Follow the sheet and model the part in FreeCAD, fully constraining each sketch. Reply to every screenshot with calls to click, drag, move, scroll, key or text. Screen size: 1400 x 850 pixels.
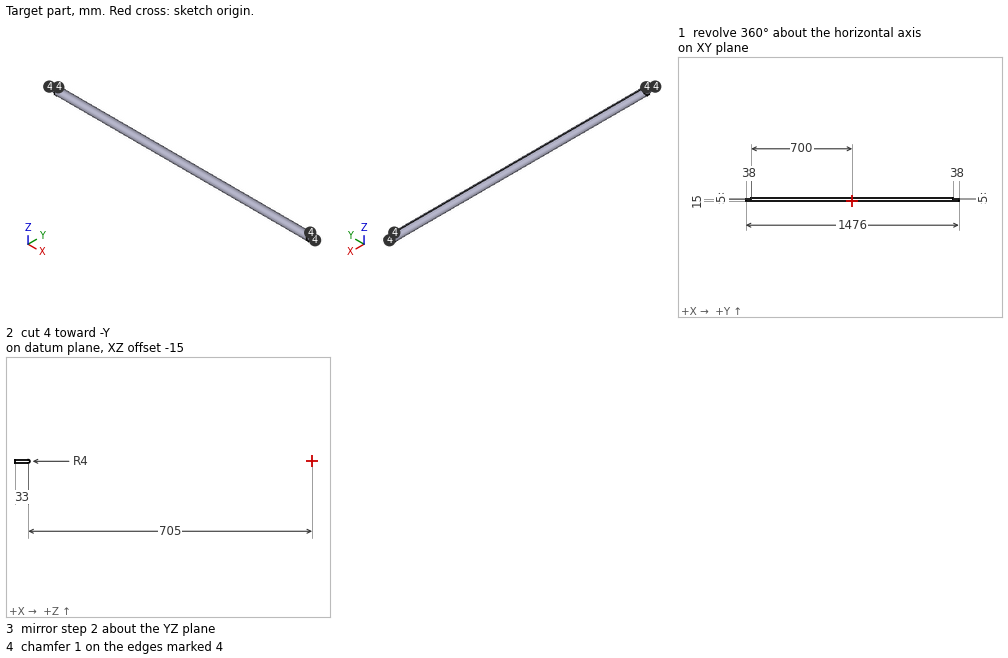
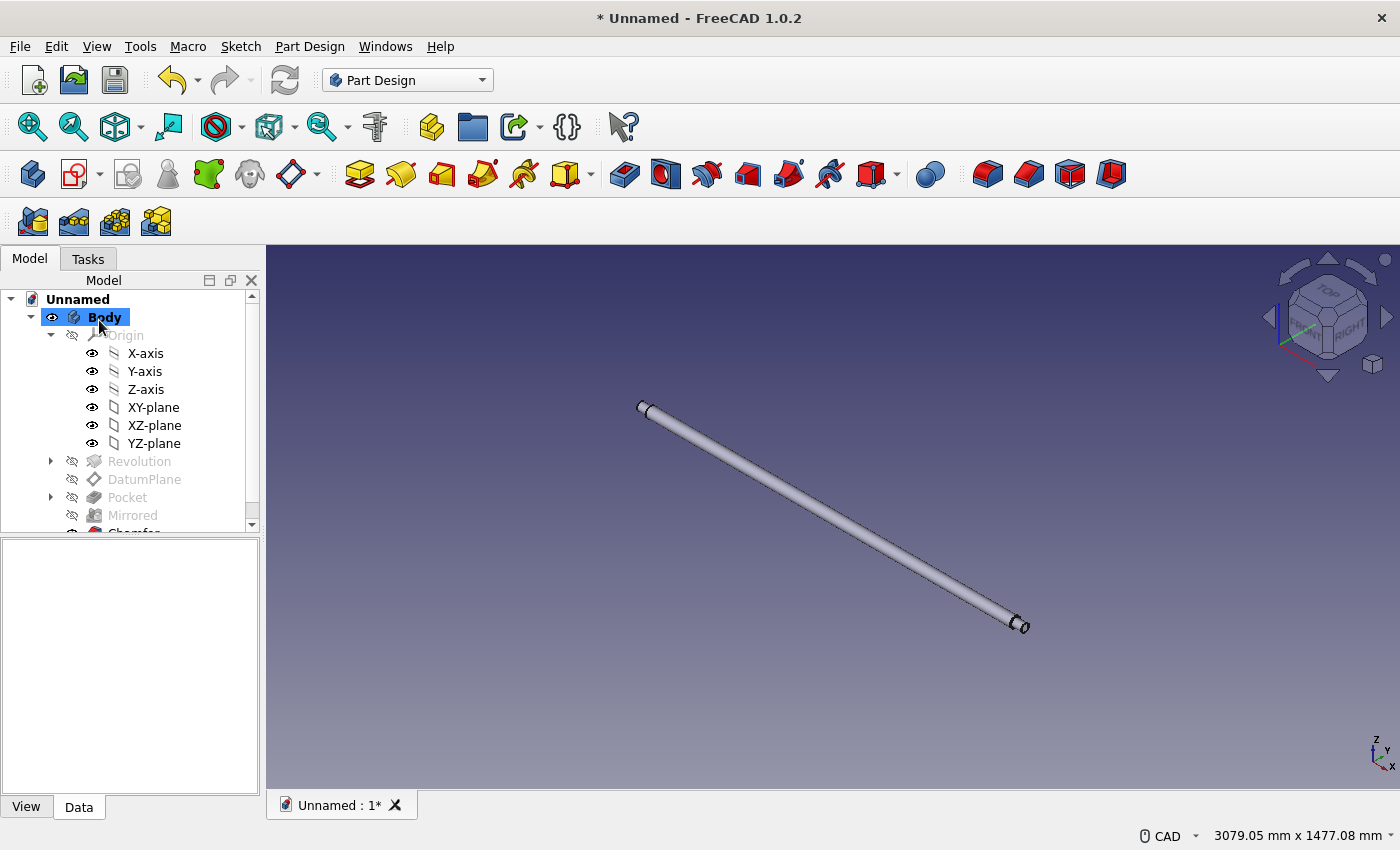
click(33, 128)